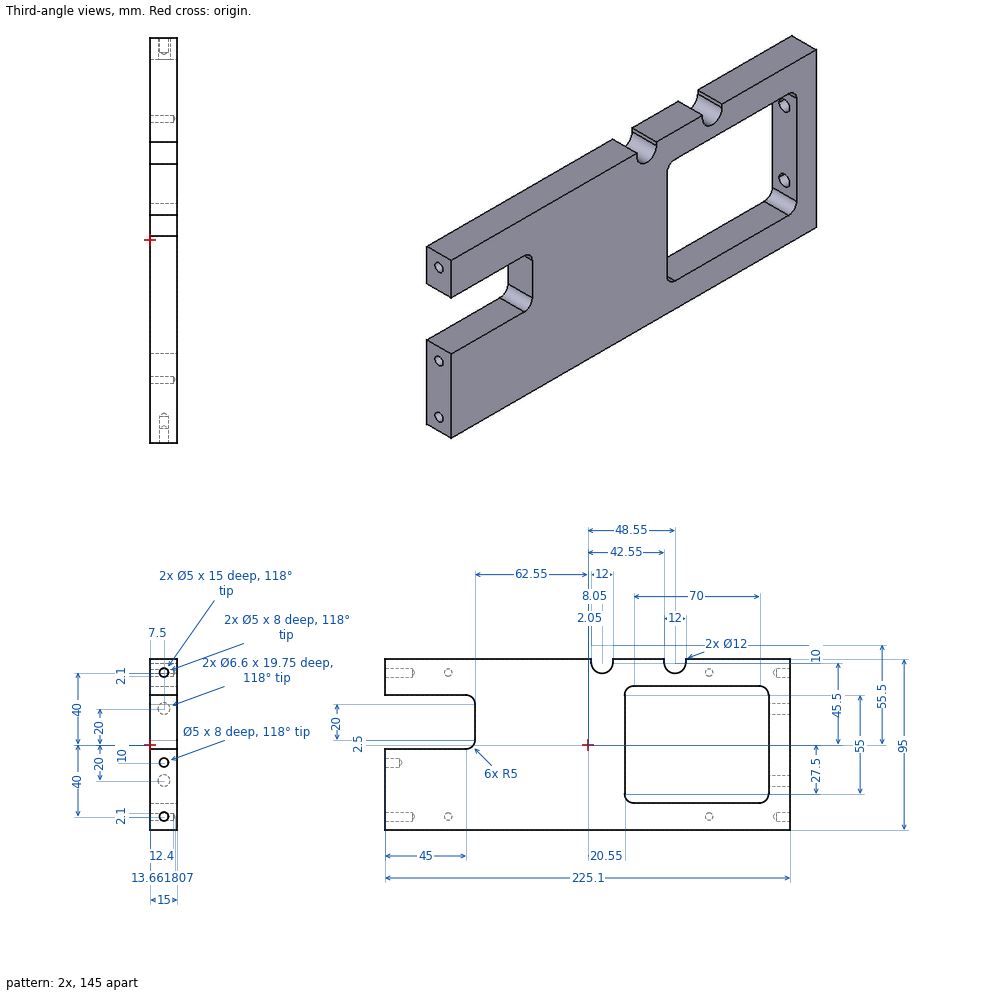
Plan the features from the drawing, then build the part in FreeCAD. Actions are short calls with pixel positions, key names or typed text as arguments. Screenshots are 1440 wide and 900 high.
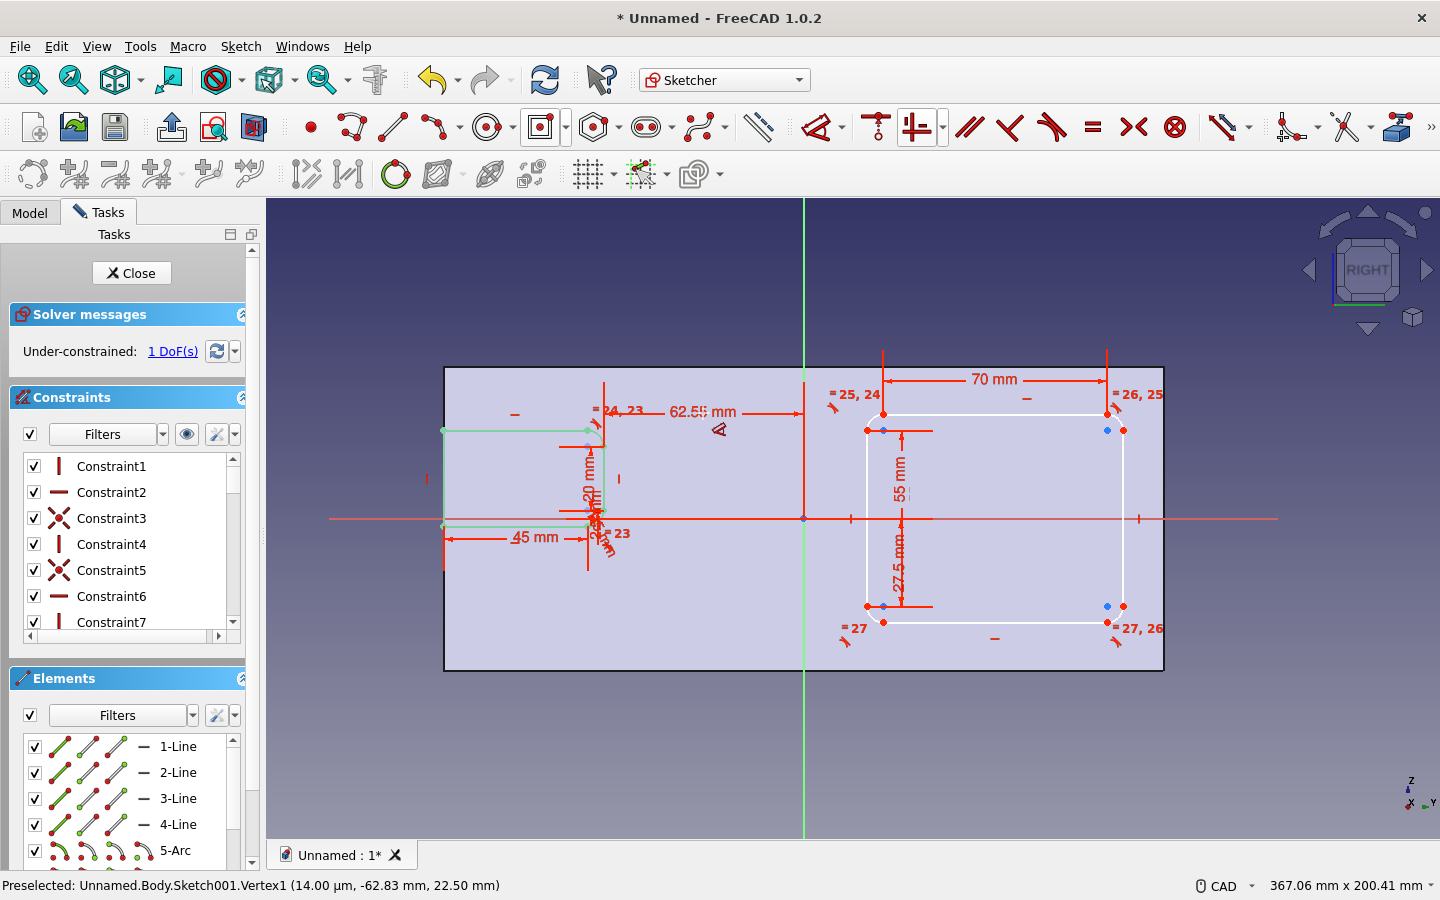
click(867, 607)
click(835, 641)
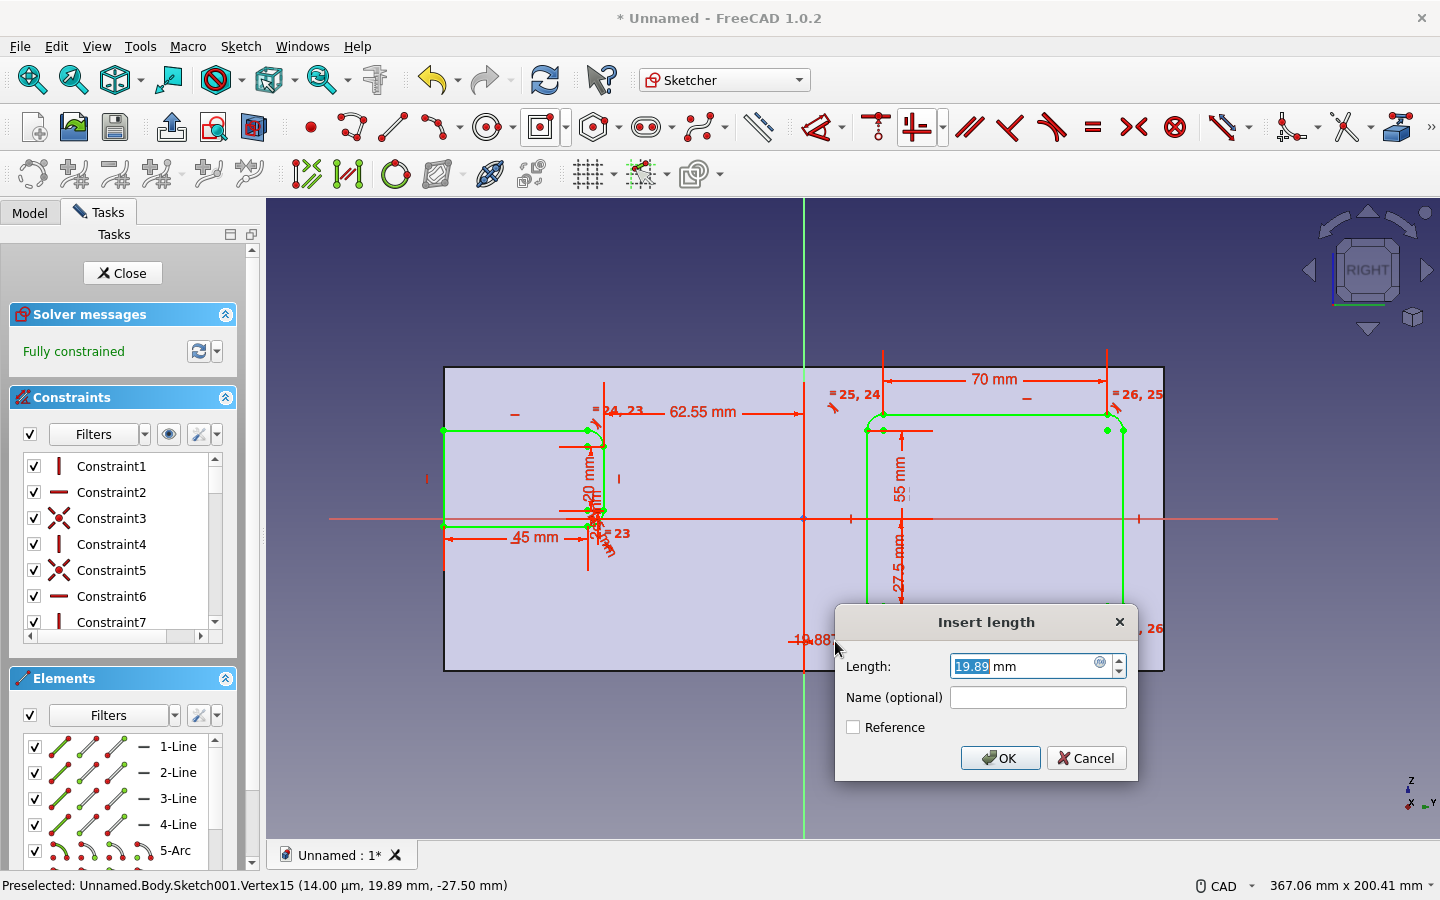
text(20.55)
key(Return)
key(Escape)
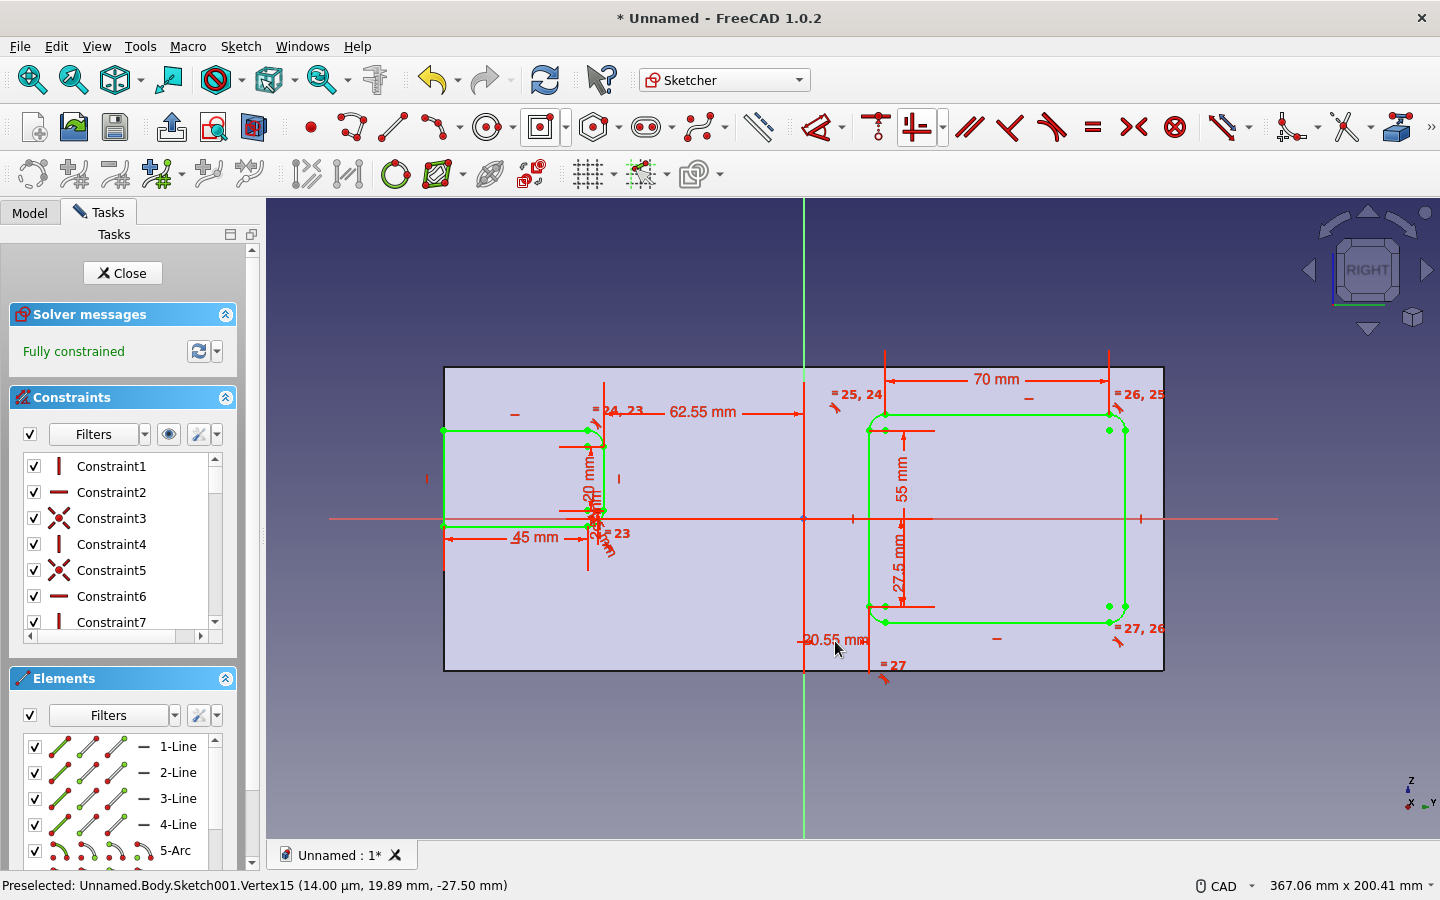
click(123, 273)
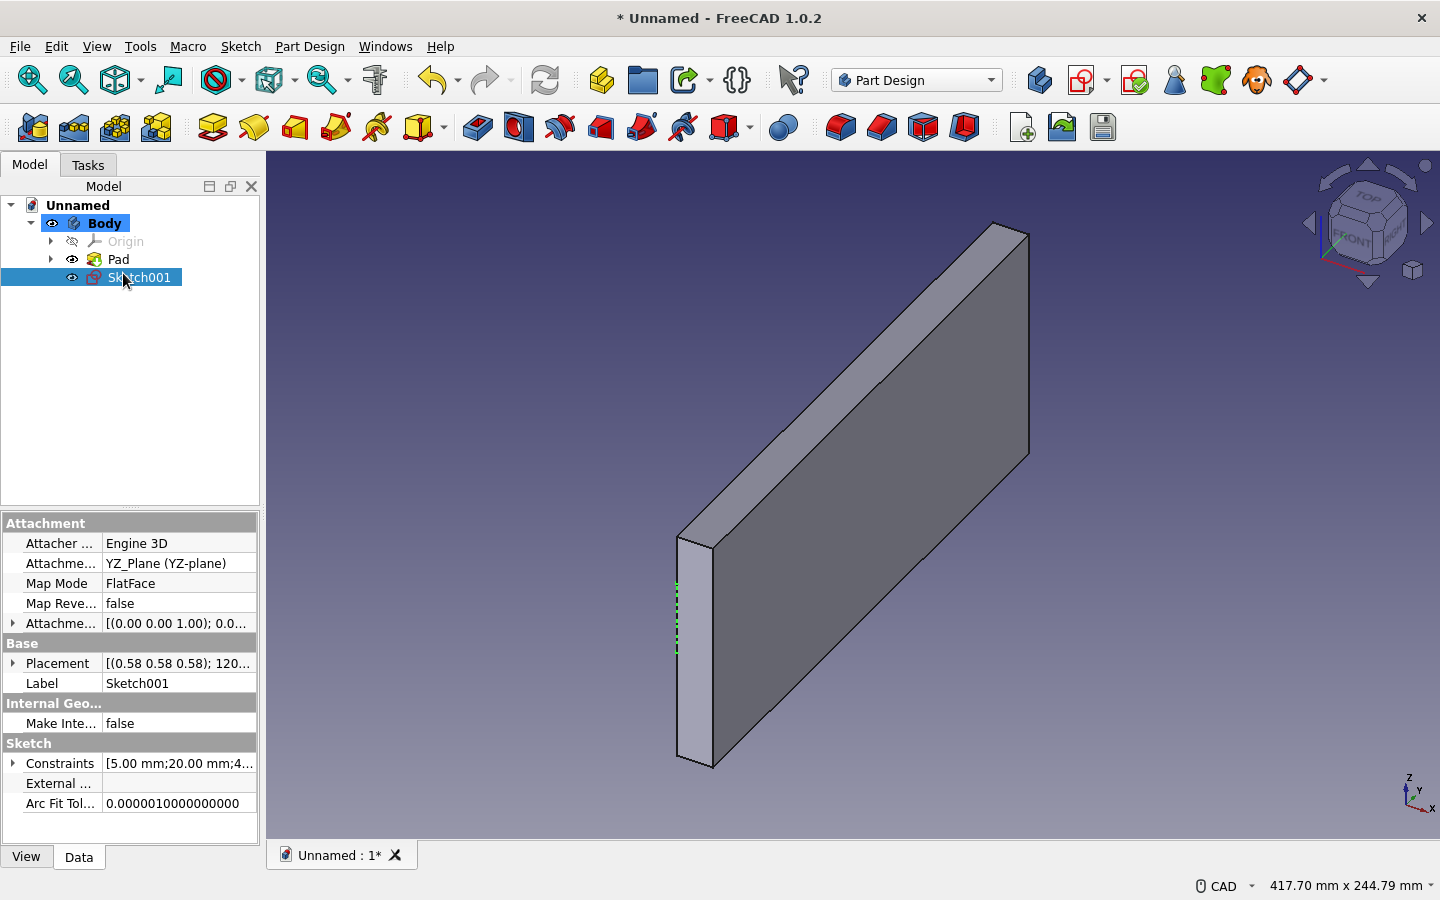
click(478, 128)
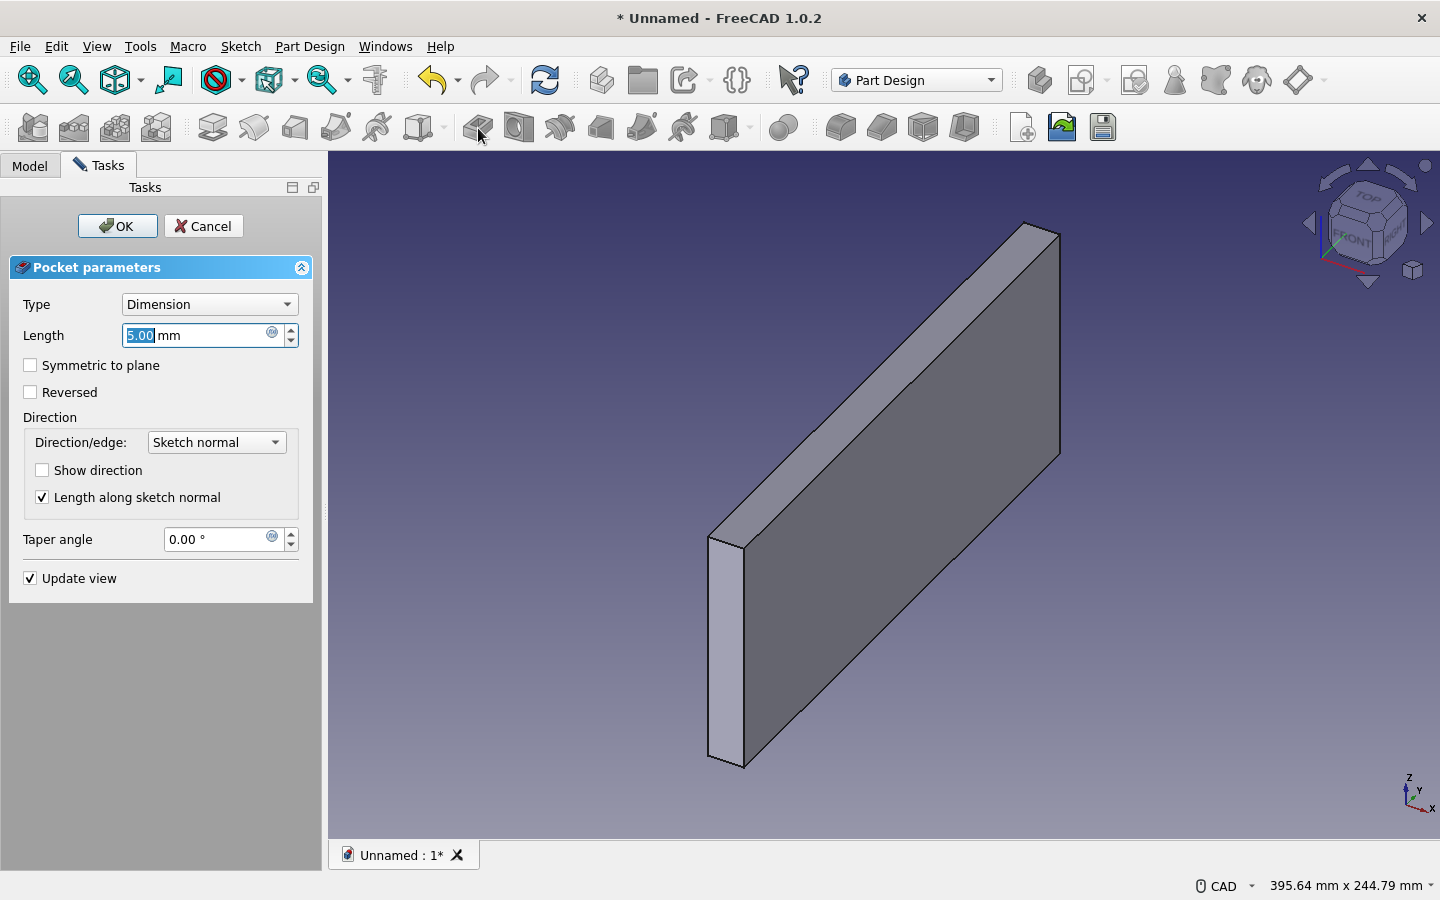
click(210, 304)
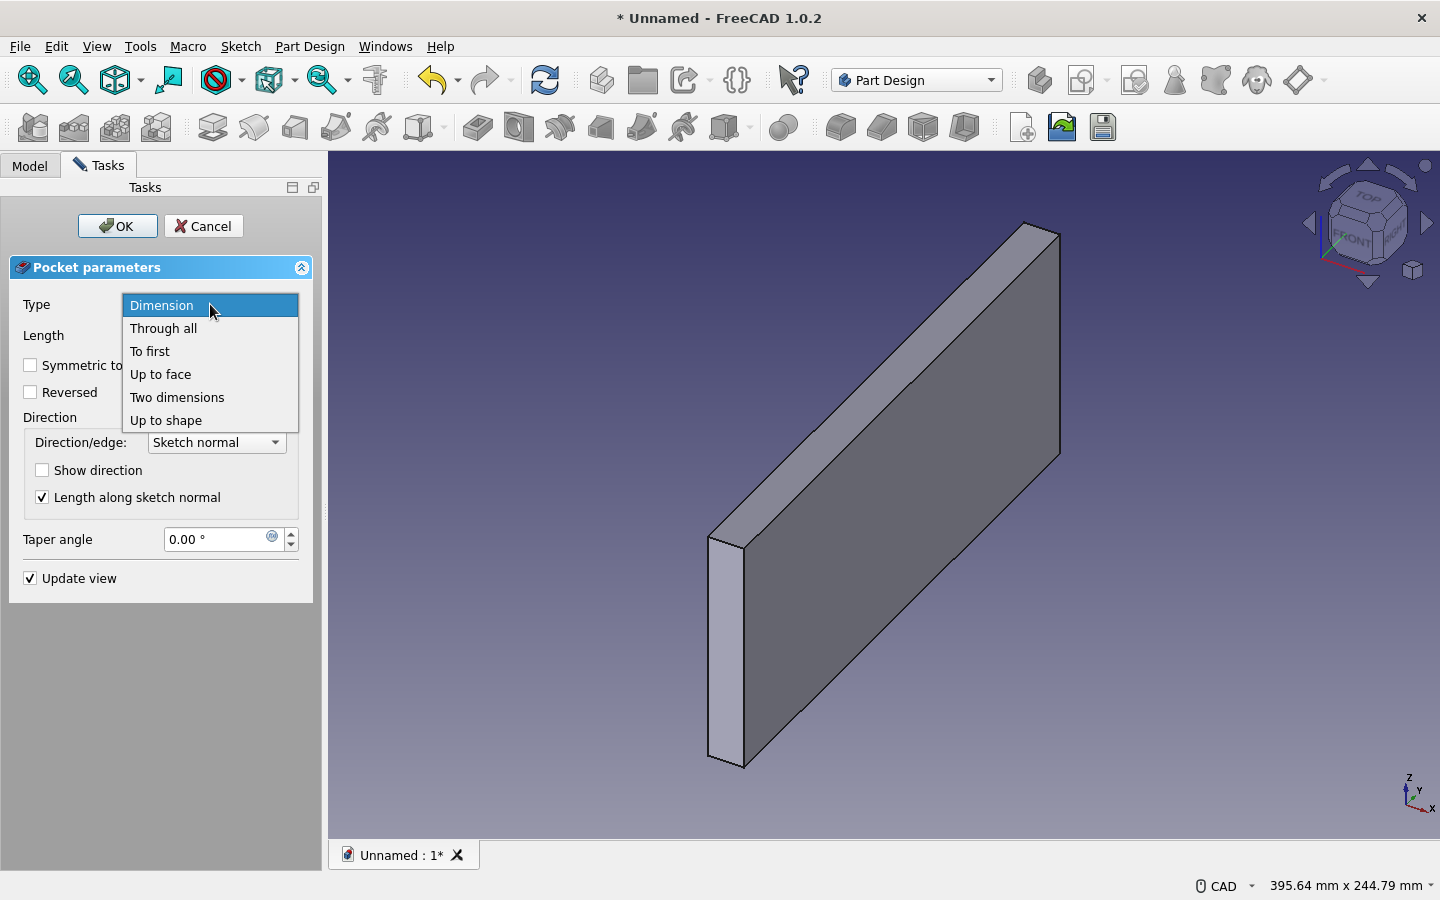
click(208, 328)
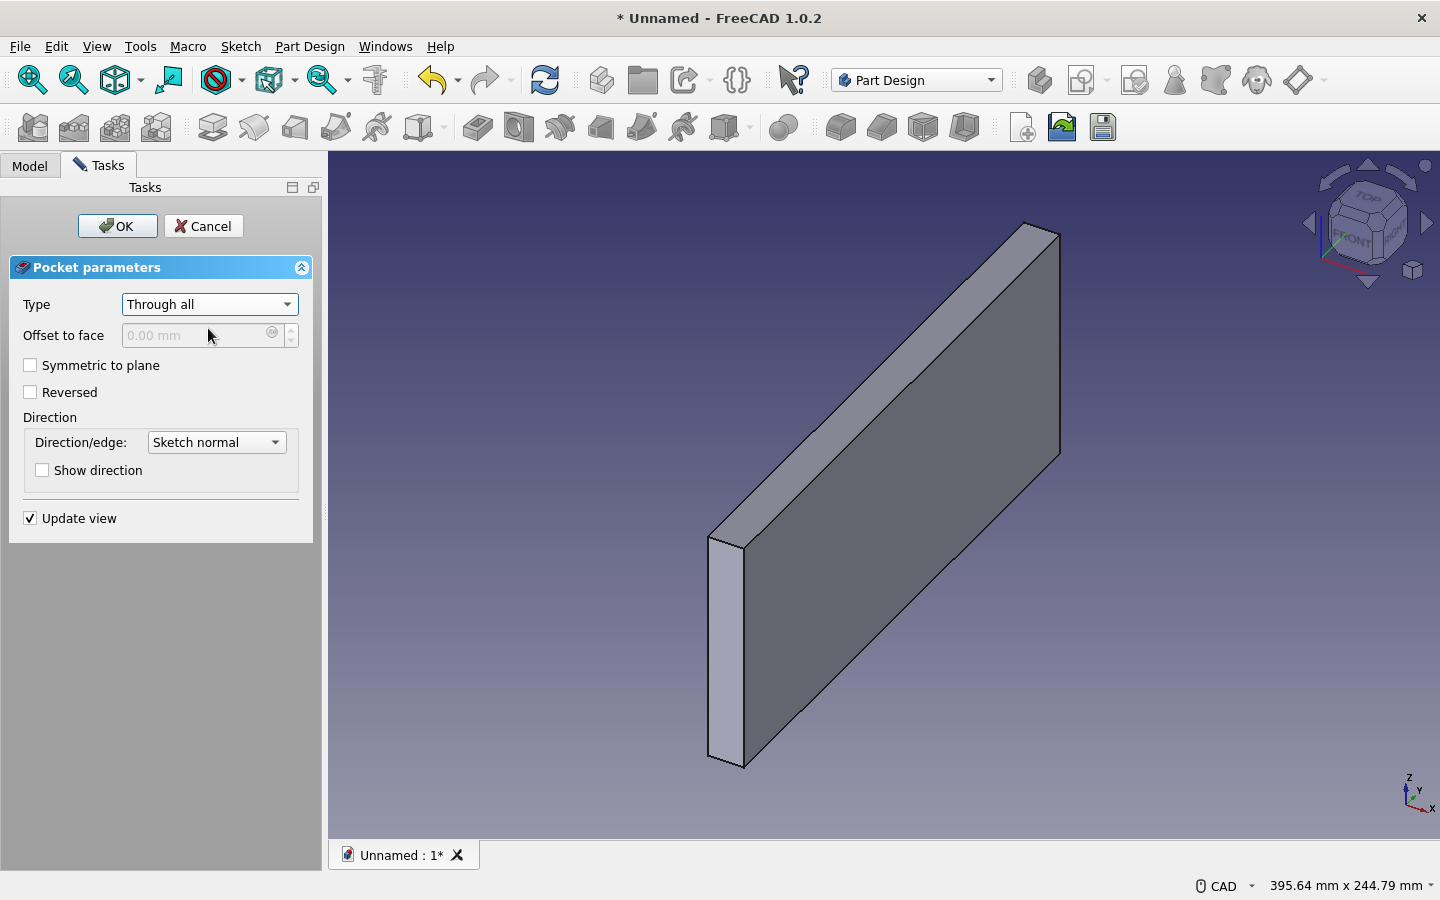
click(31, 392)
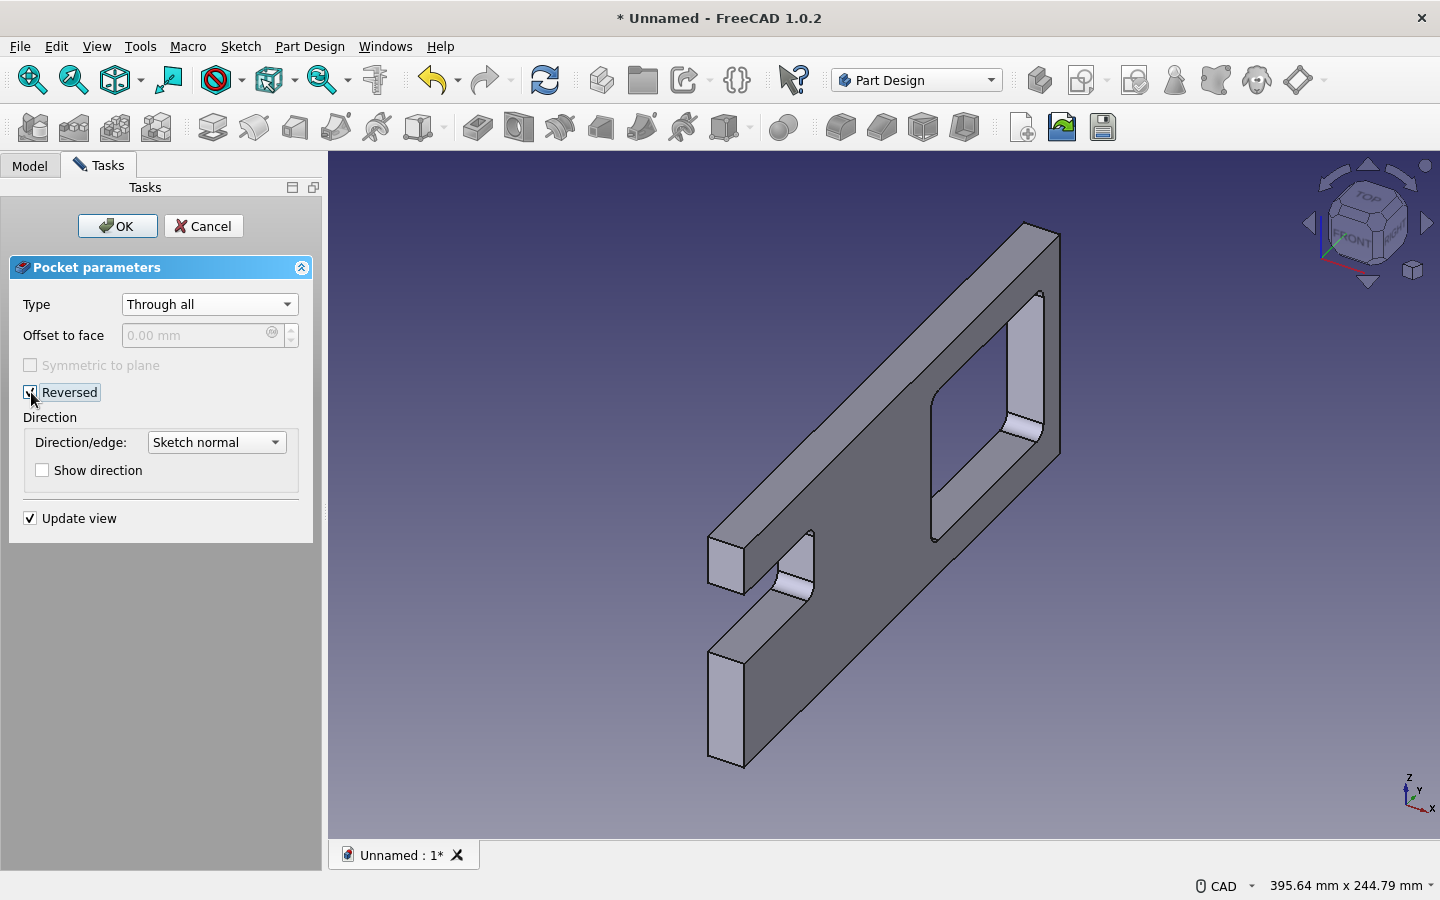
click(118, 226)